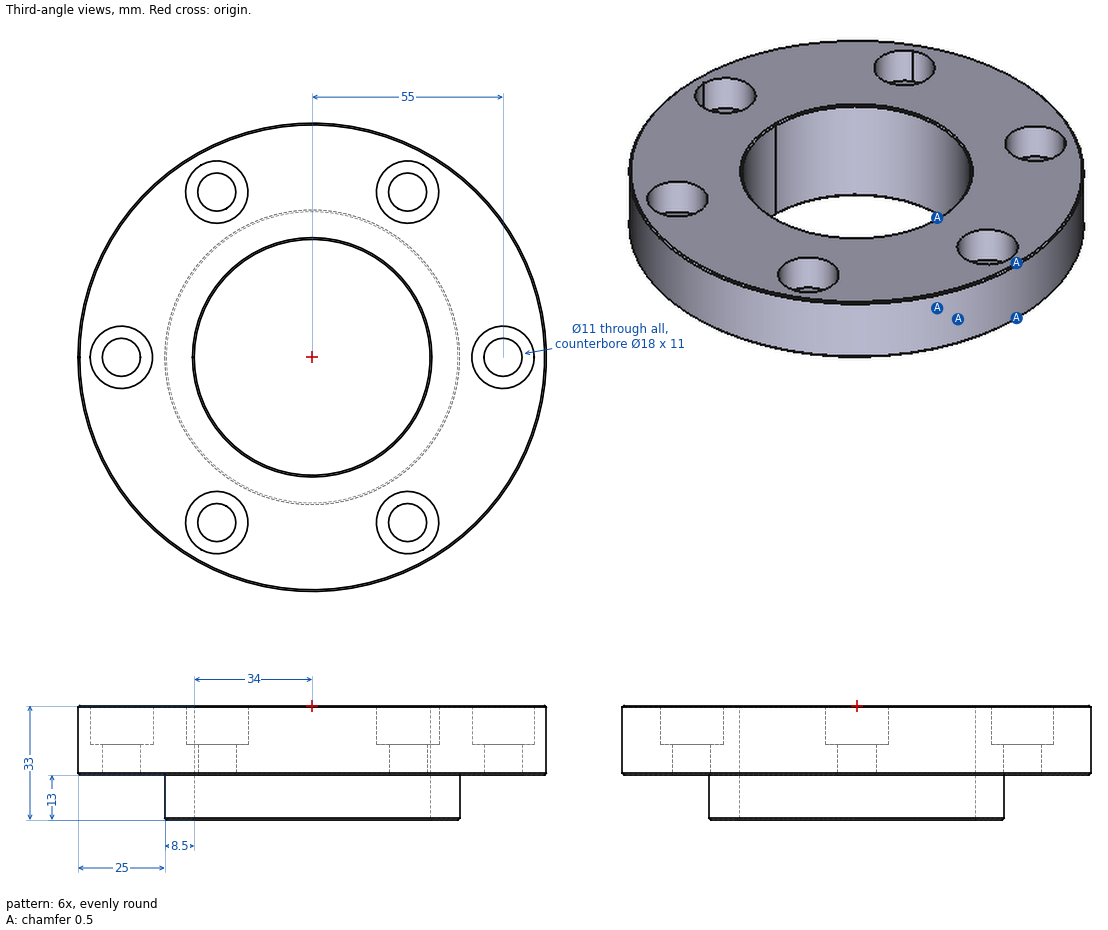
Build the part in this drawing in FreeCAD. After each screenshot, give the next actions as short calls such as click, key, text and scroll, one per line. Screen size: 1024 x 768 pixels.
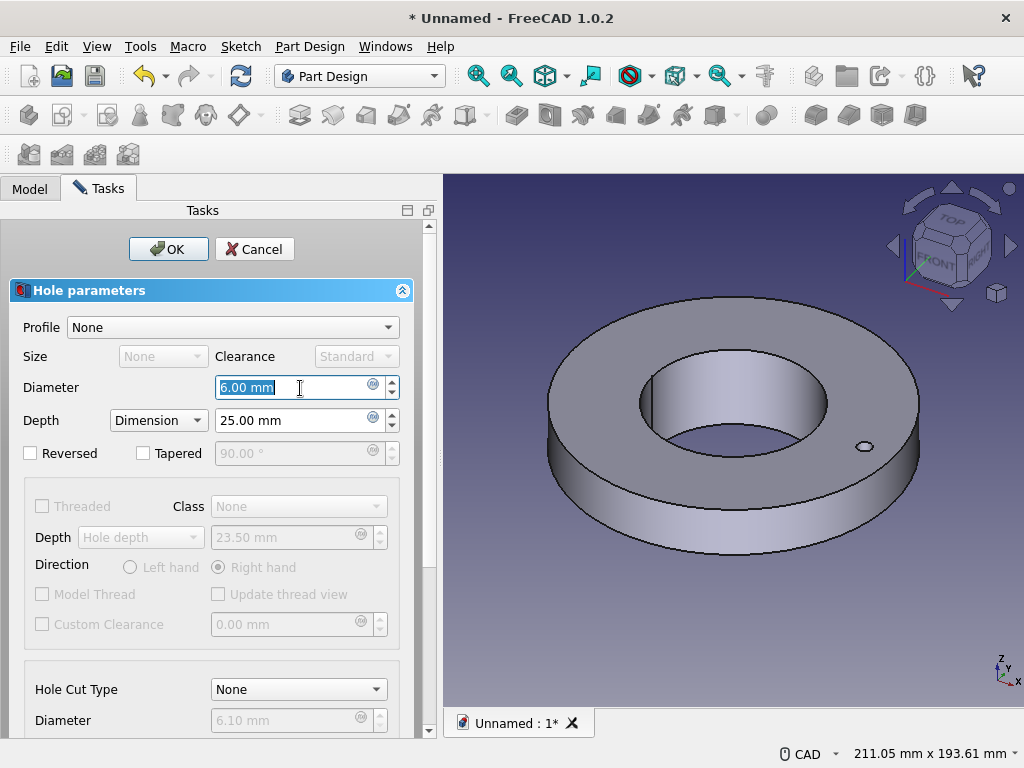
text(11)
key(Tab)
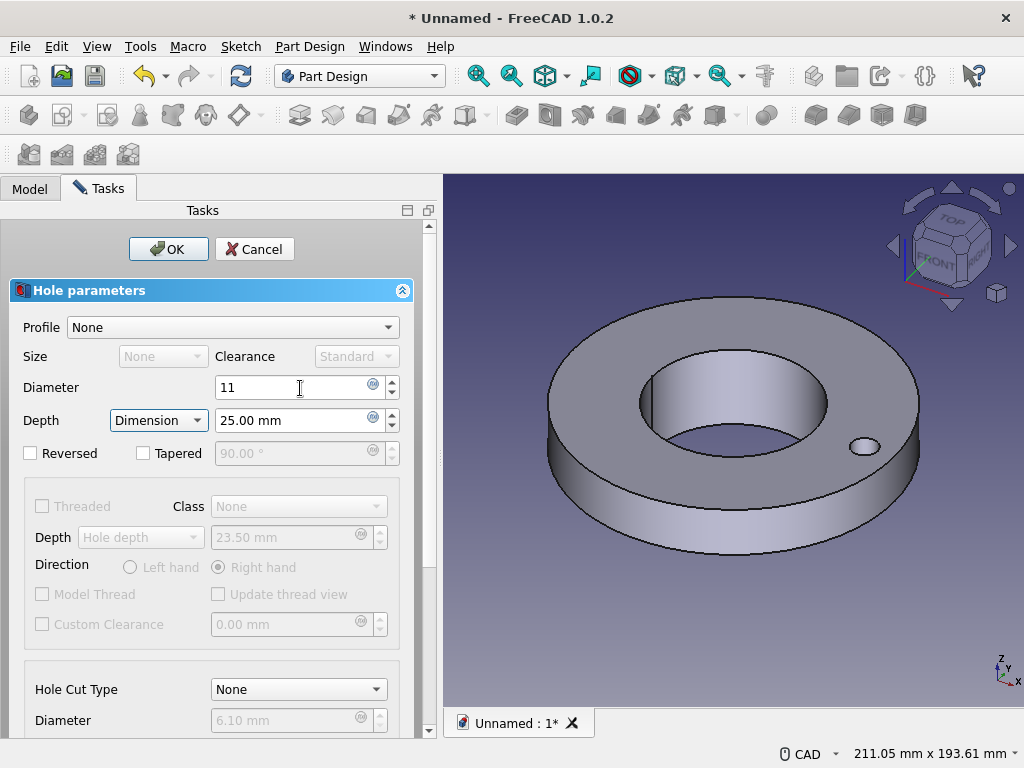
click(160, 420)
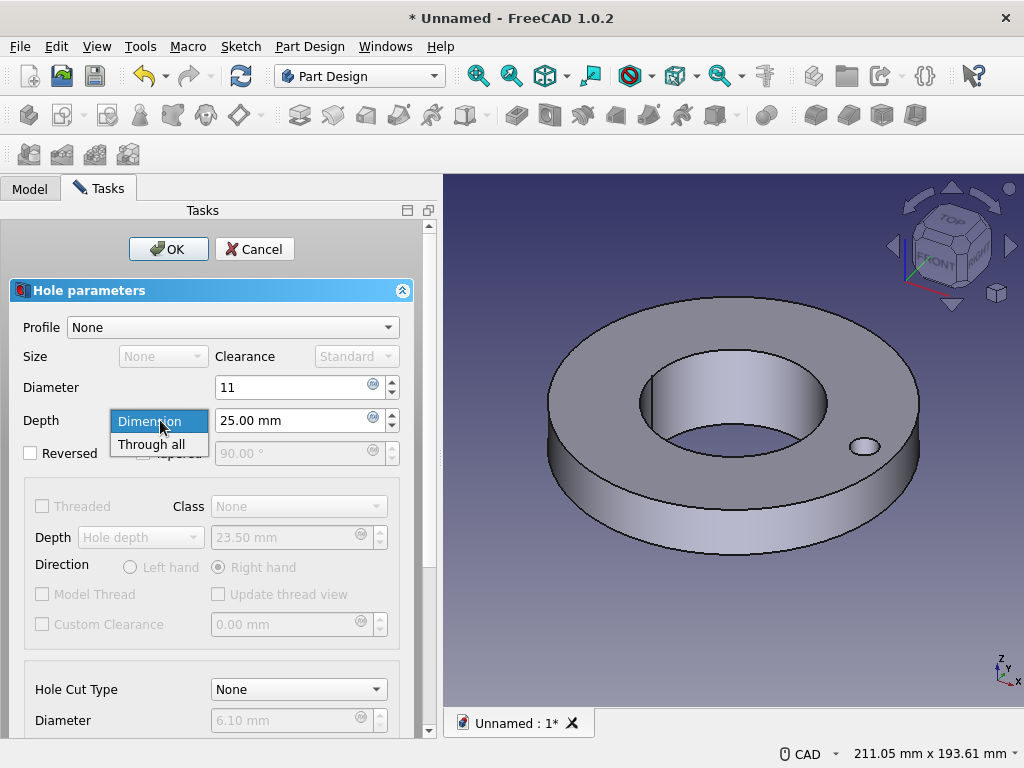
click(158, 444)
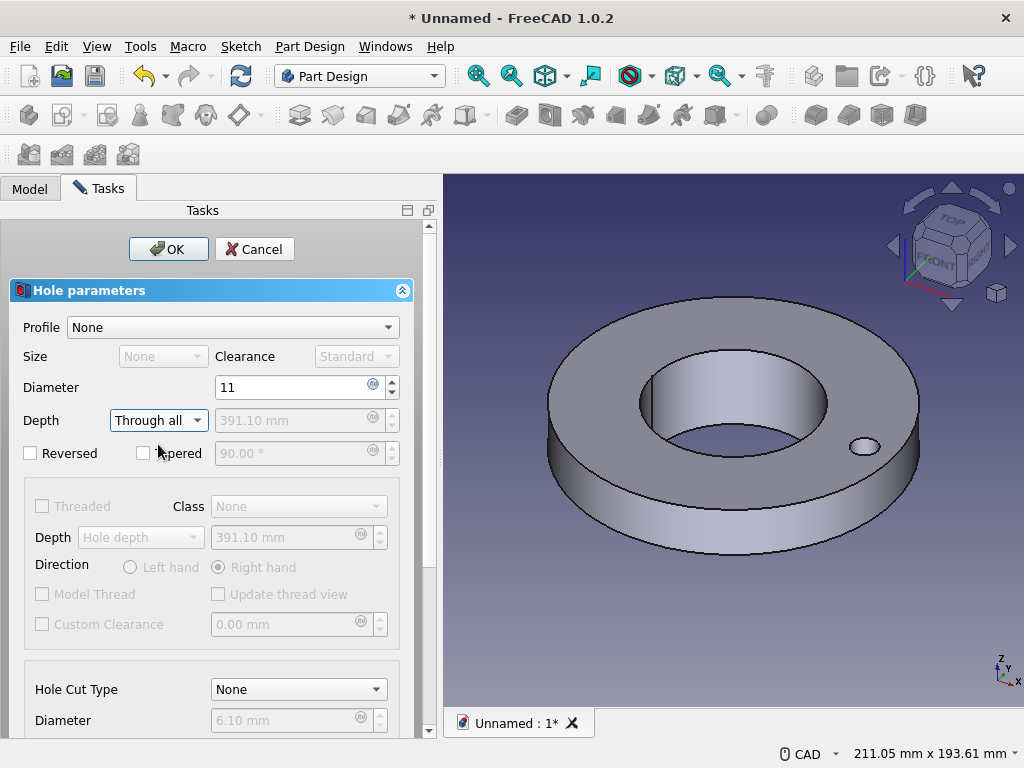
click(300, 690)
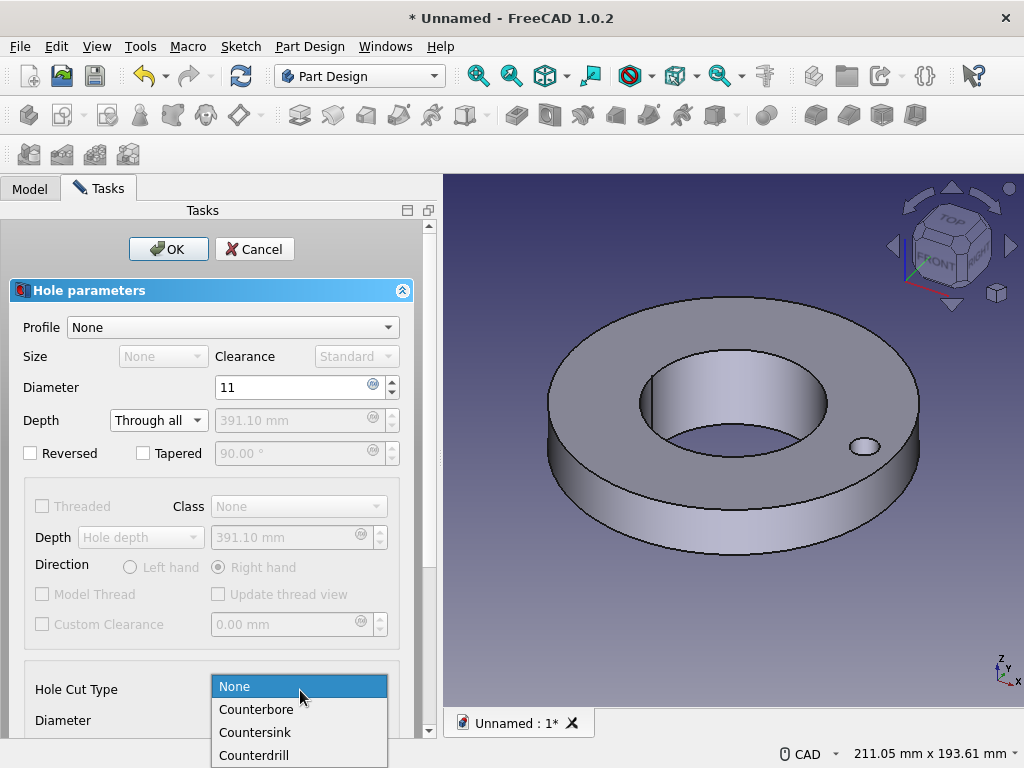
click(298, 710)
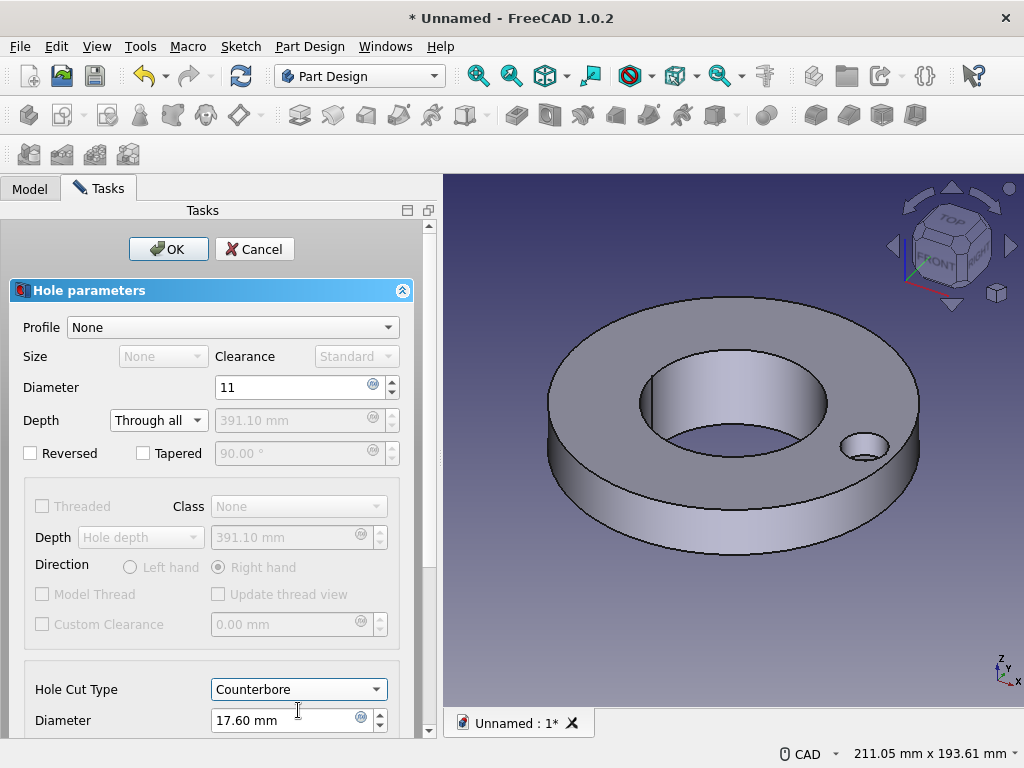
triple_click(292, 720)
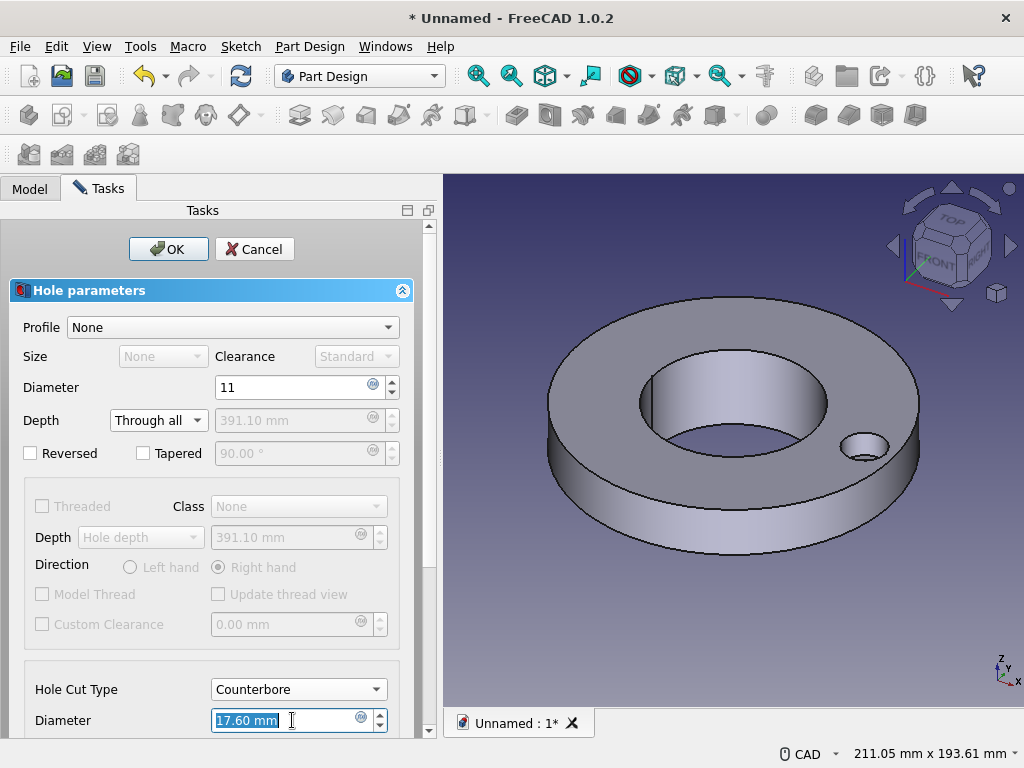
text(18)
key(Tab)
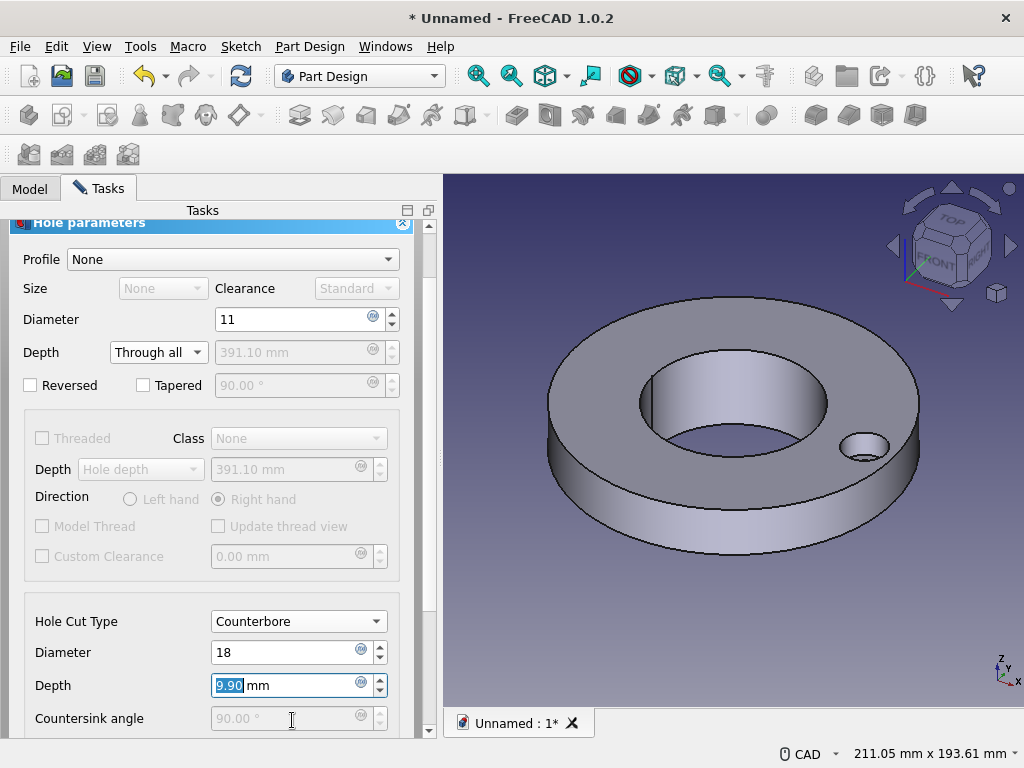
text(11)
key(Tab)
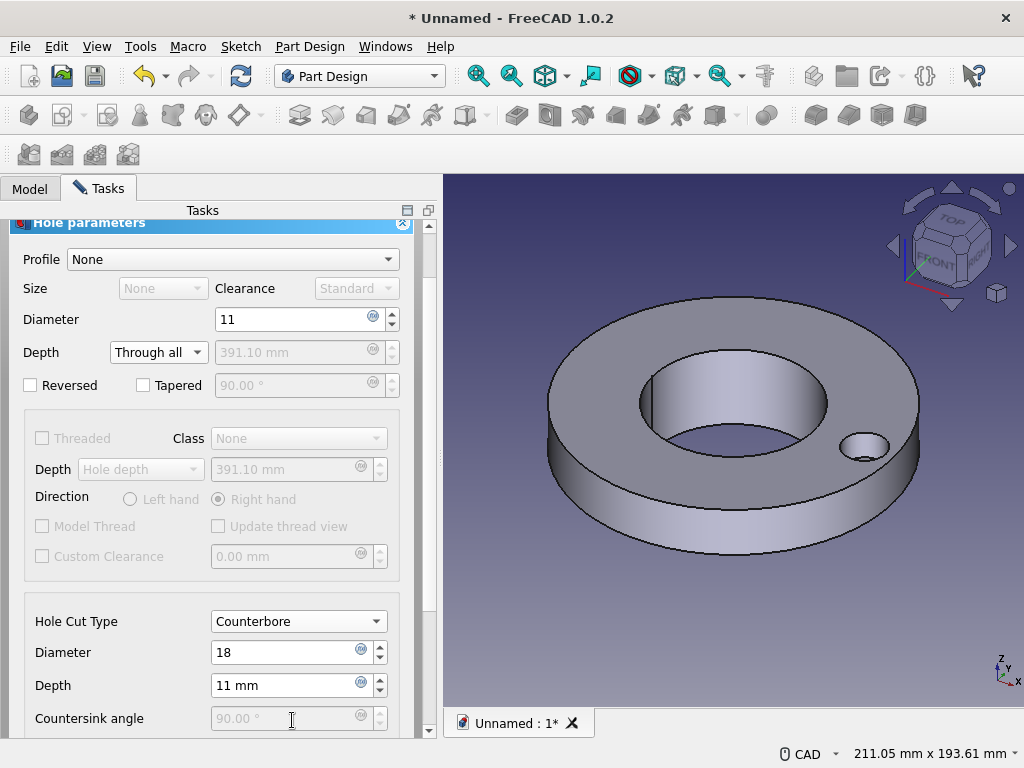
scroll(429, 479, up, 2)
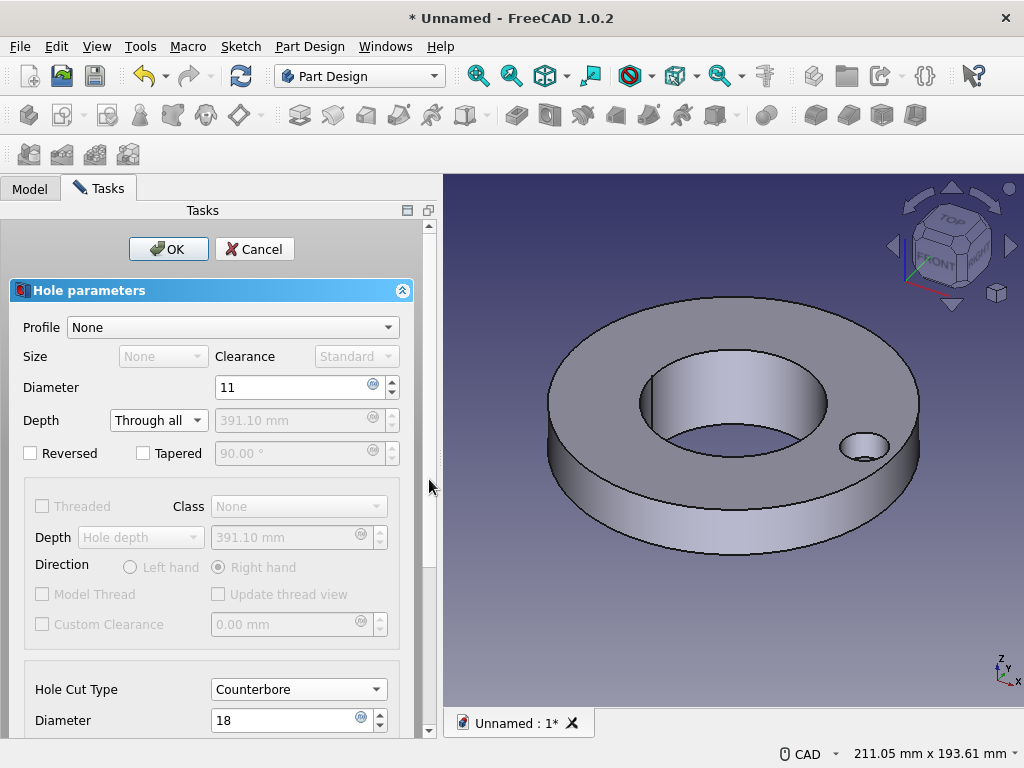
click(169, 249)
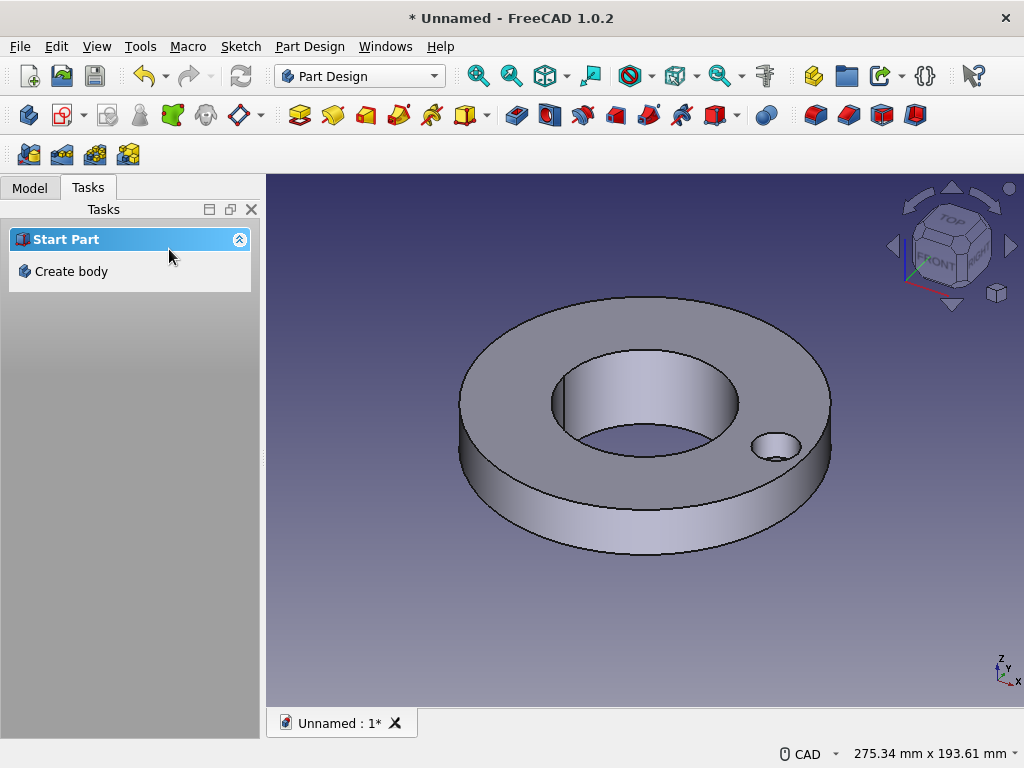
click(30, 188)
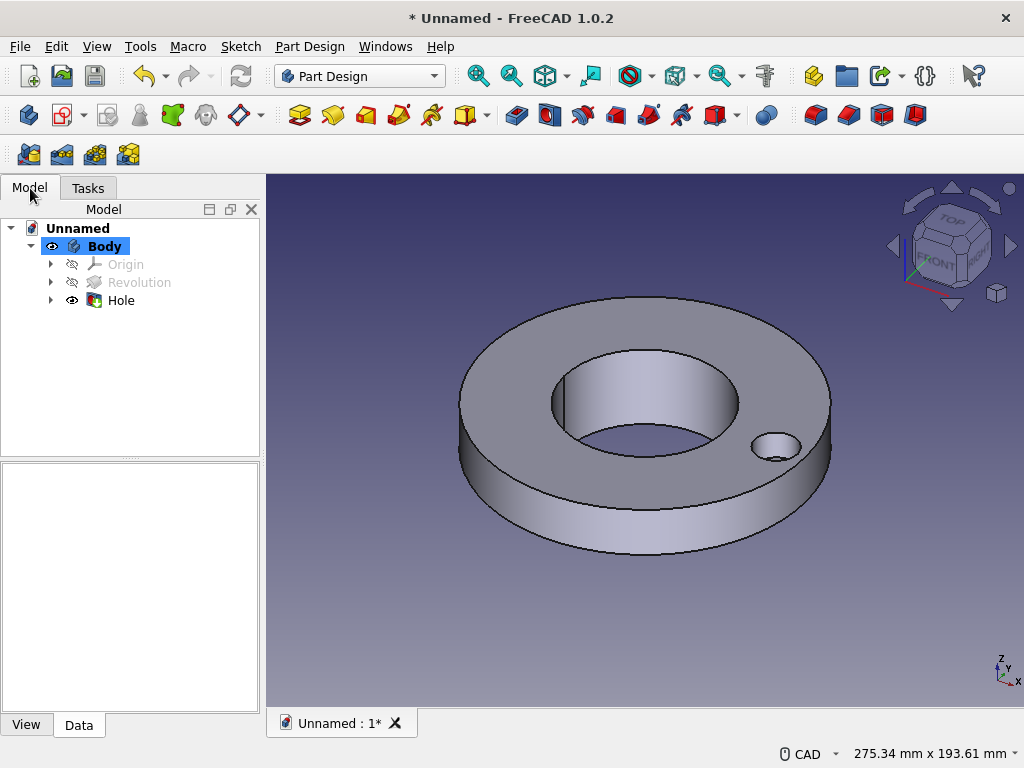
click(117, 300)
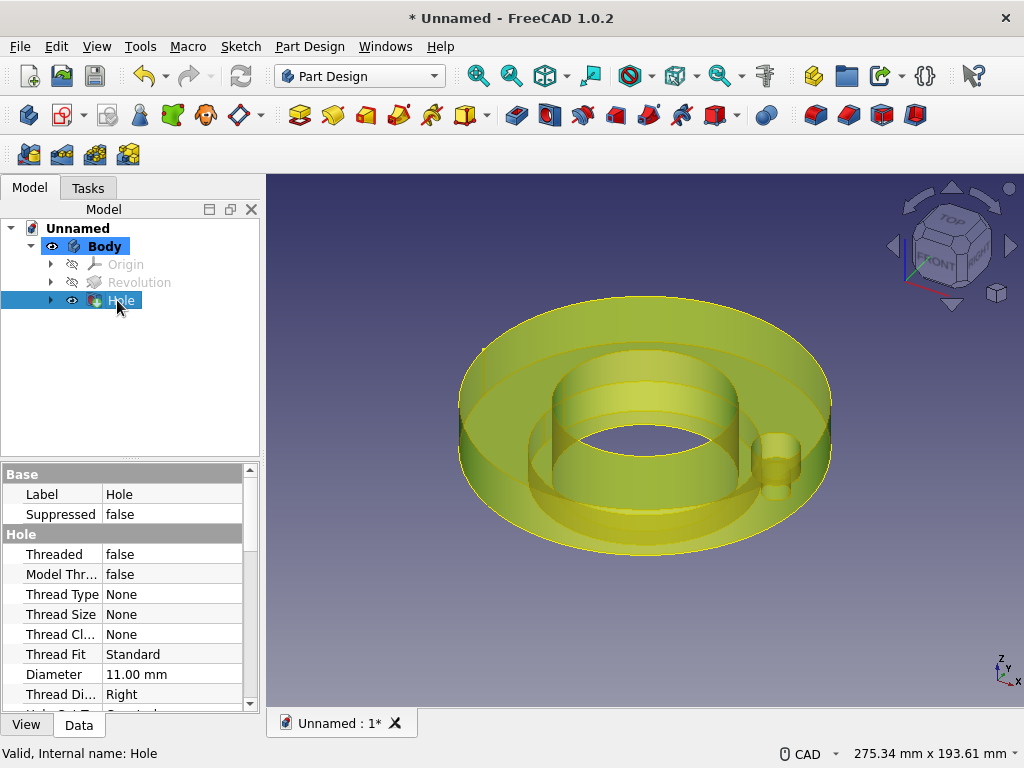
click(95, 154)